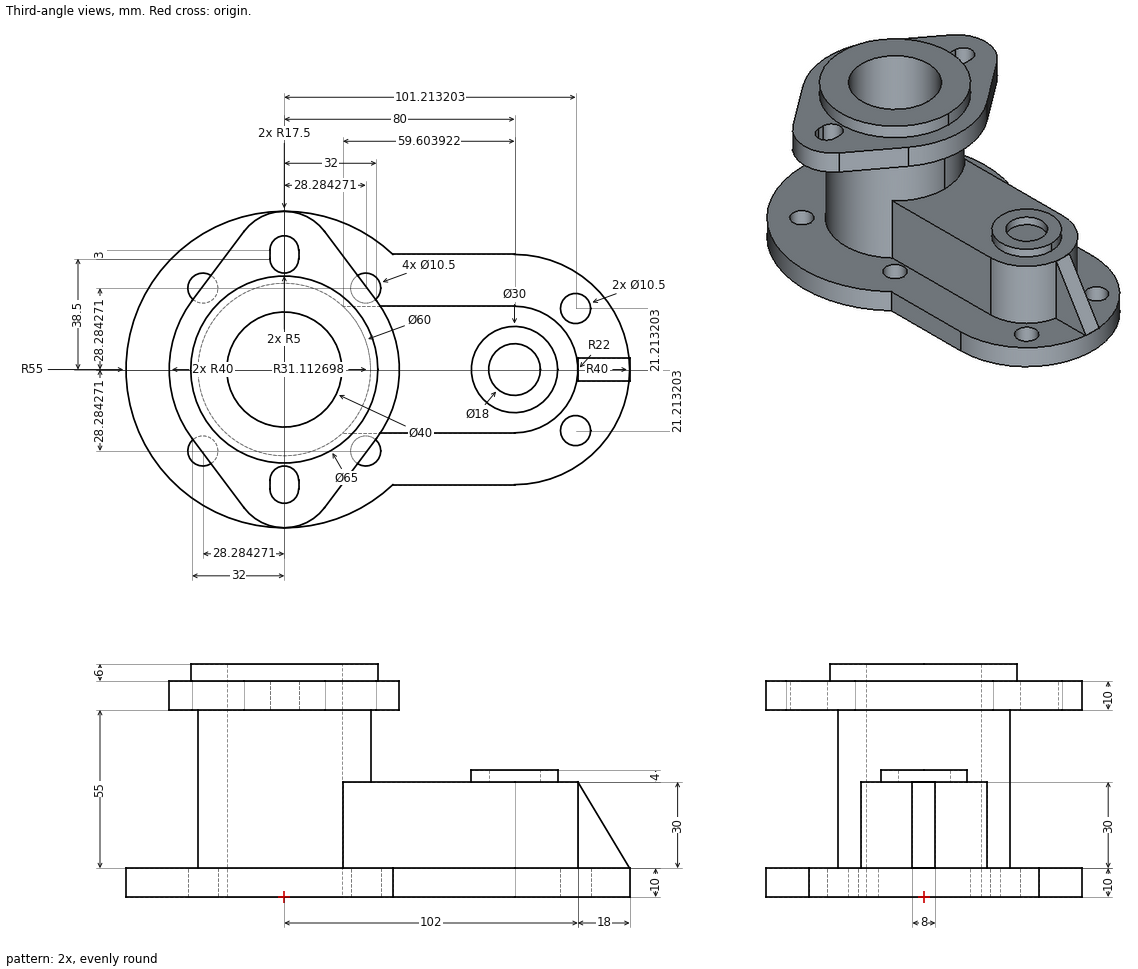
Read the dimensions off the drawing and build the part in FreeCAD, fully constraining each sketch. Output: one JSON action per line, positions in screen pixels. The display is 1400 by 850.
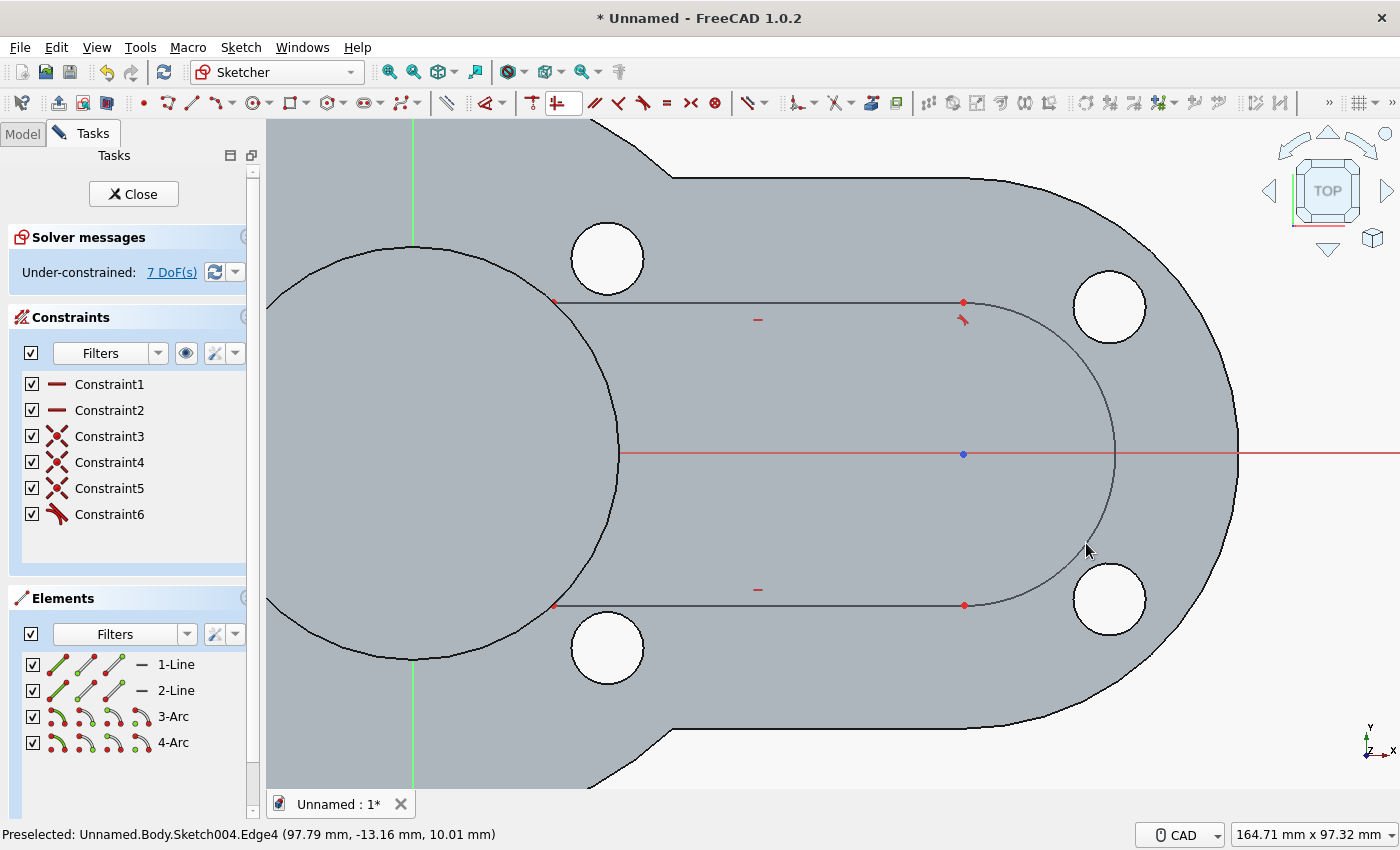
{"action": "left_click", "coordinate": [676, 606]}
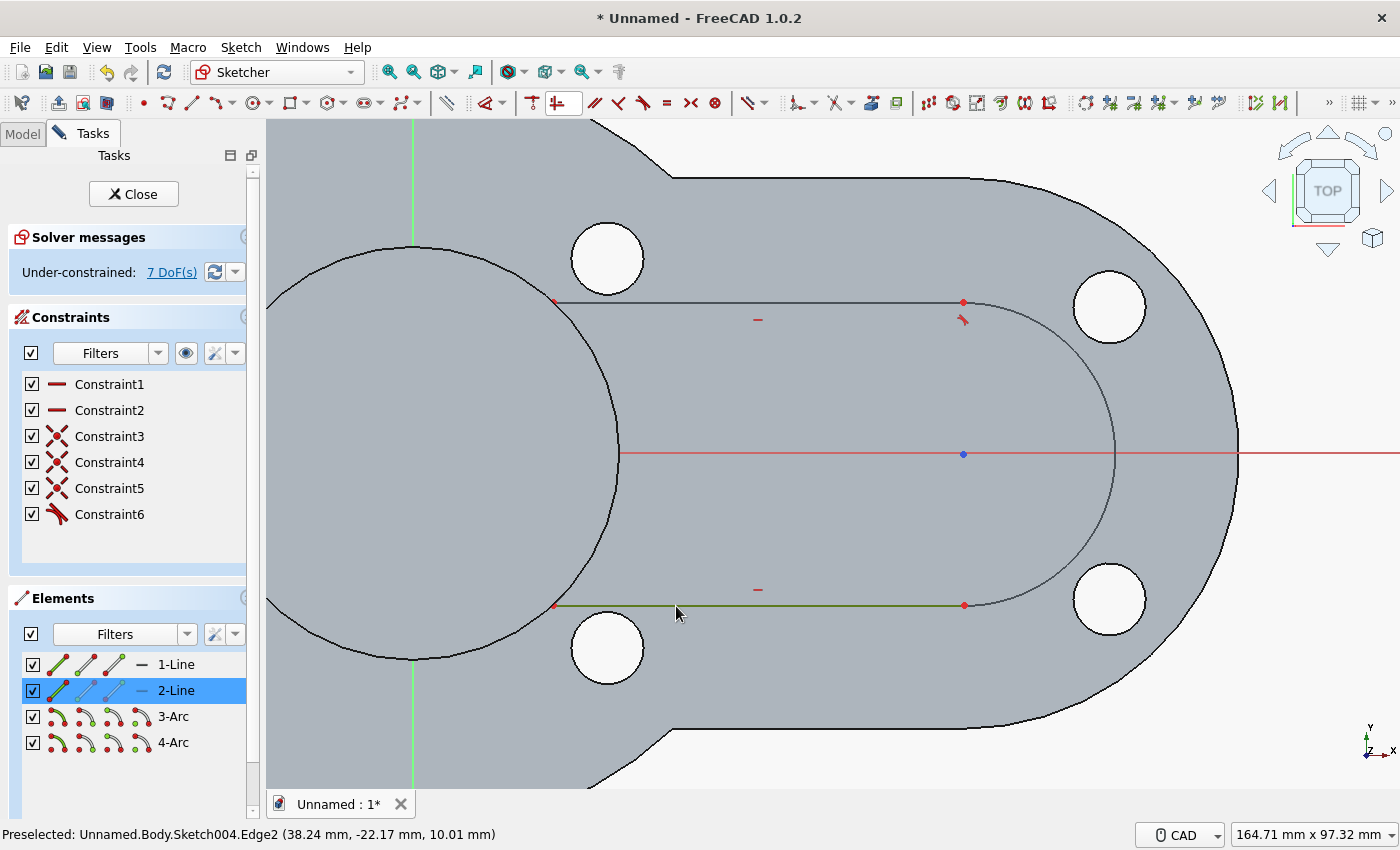
{"action": "left_click", "coordinate": [1086, 543]}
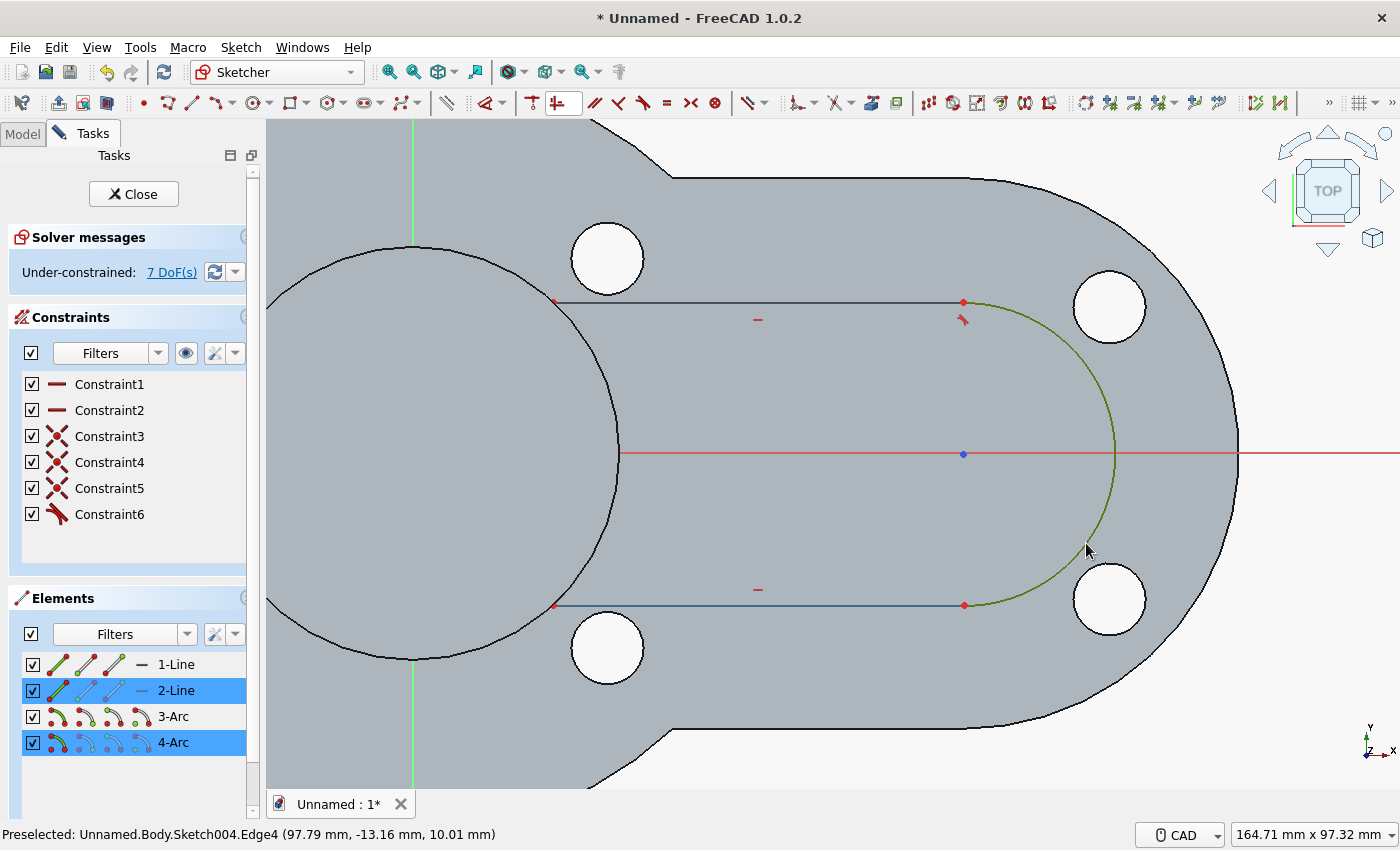
{"action": "left_click", "coordinate": [644, 104]}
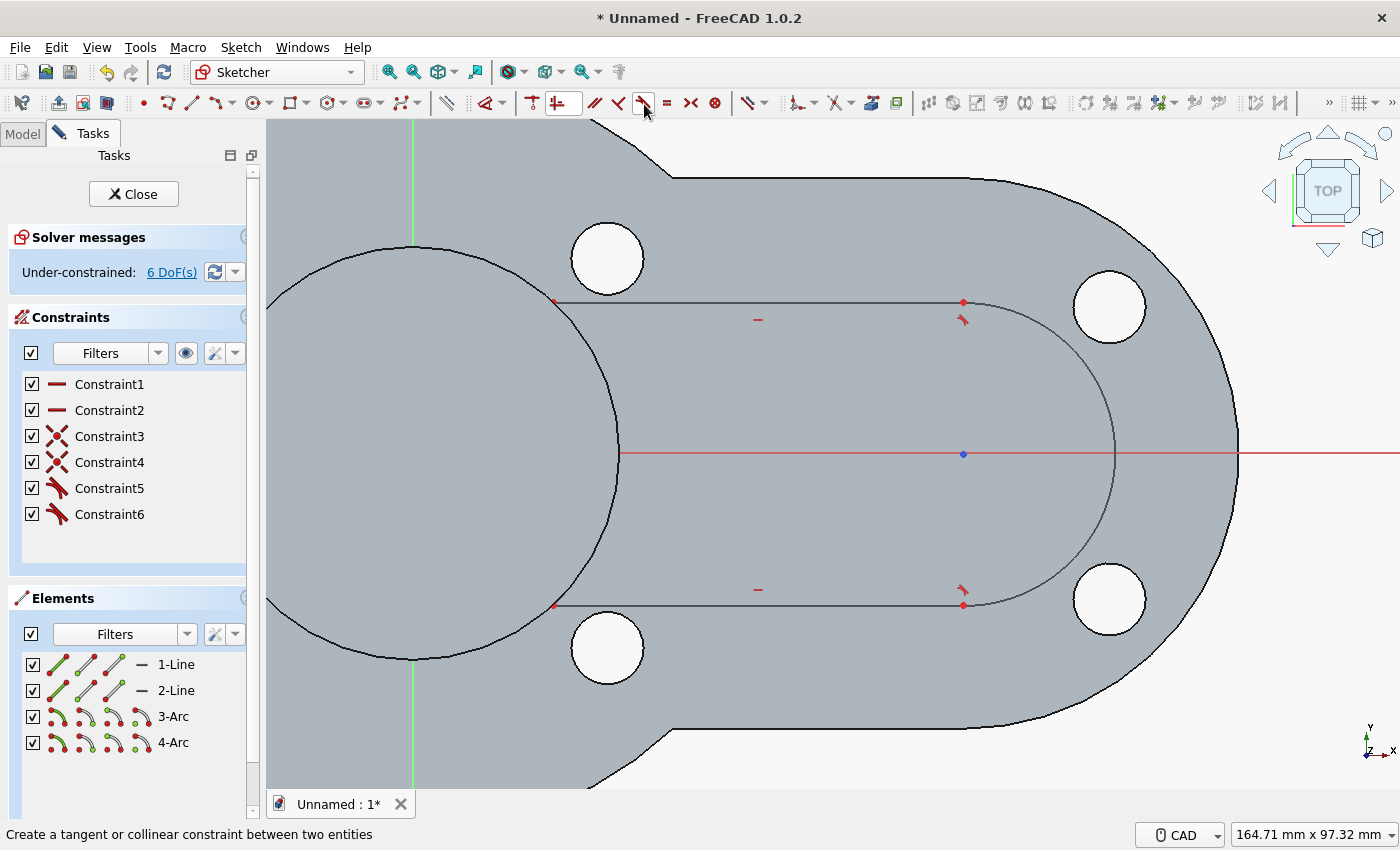
{"action": "left_click", "coordinate": [401, 454]}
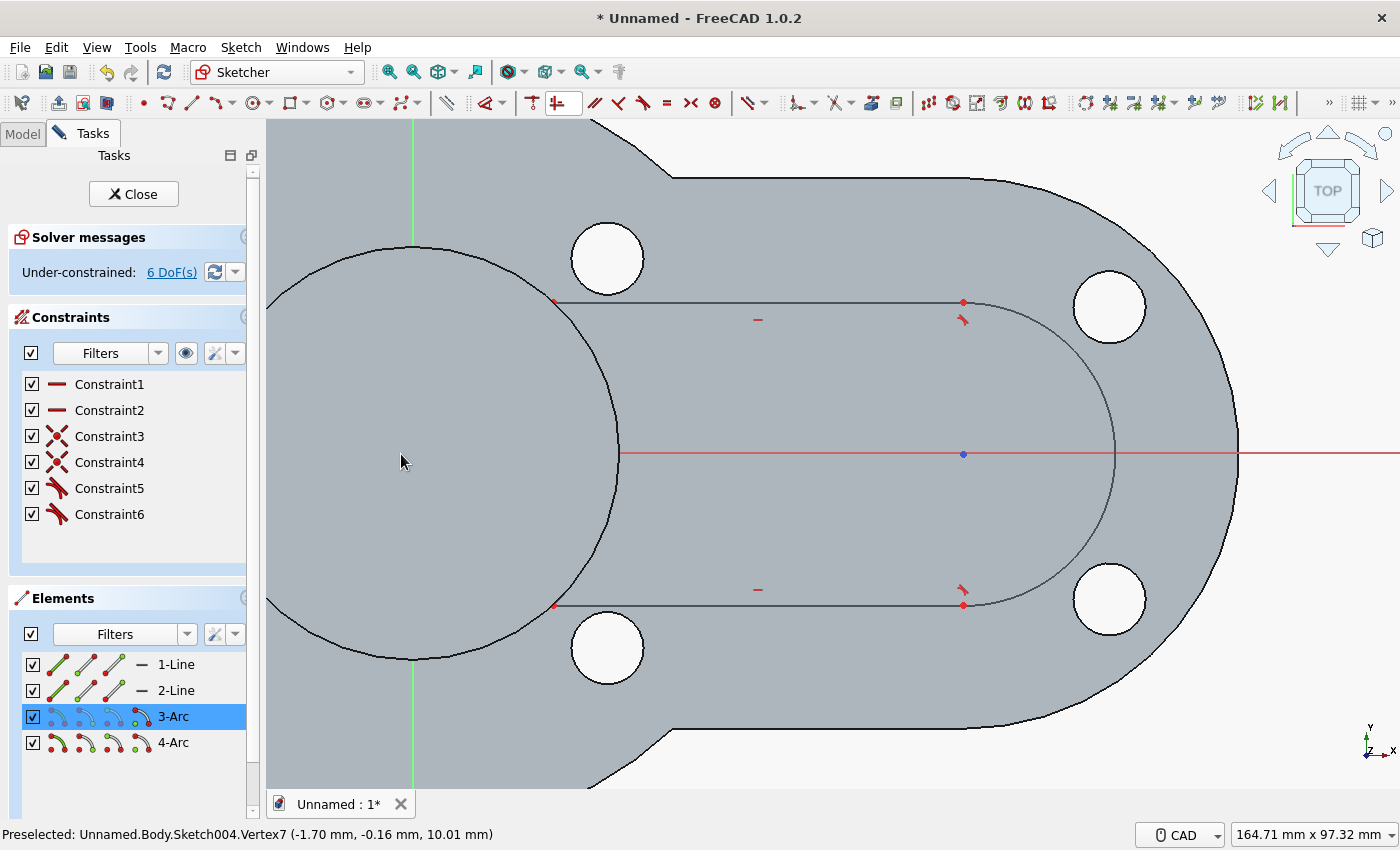
{"action": "left_click", "coordinate": [361, 453]}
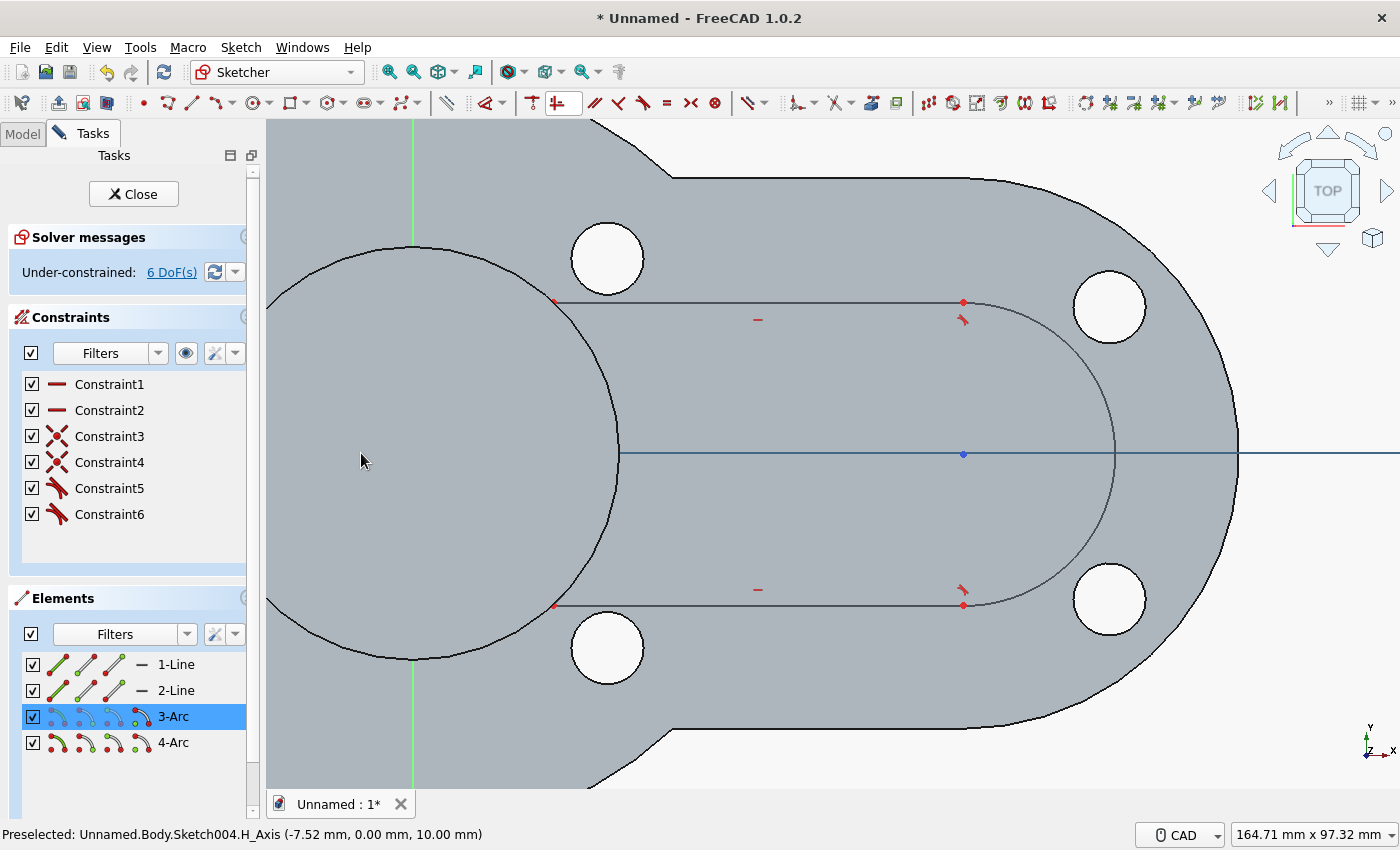
{"action": "key", "text": "c"}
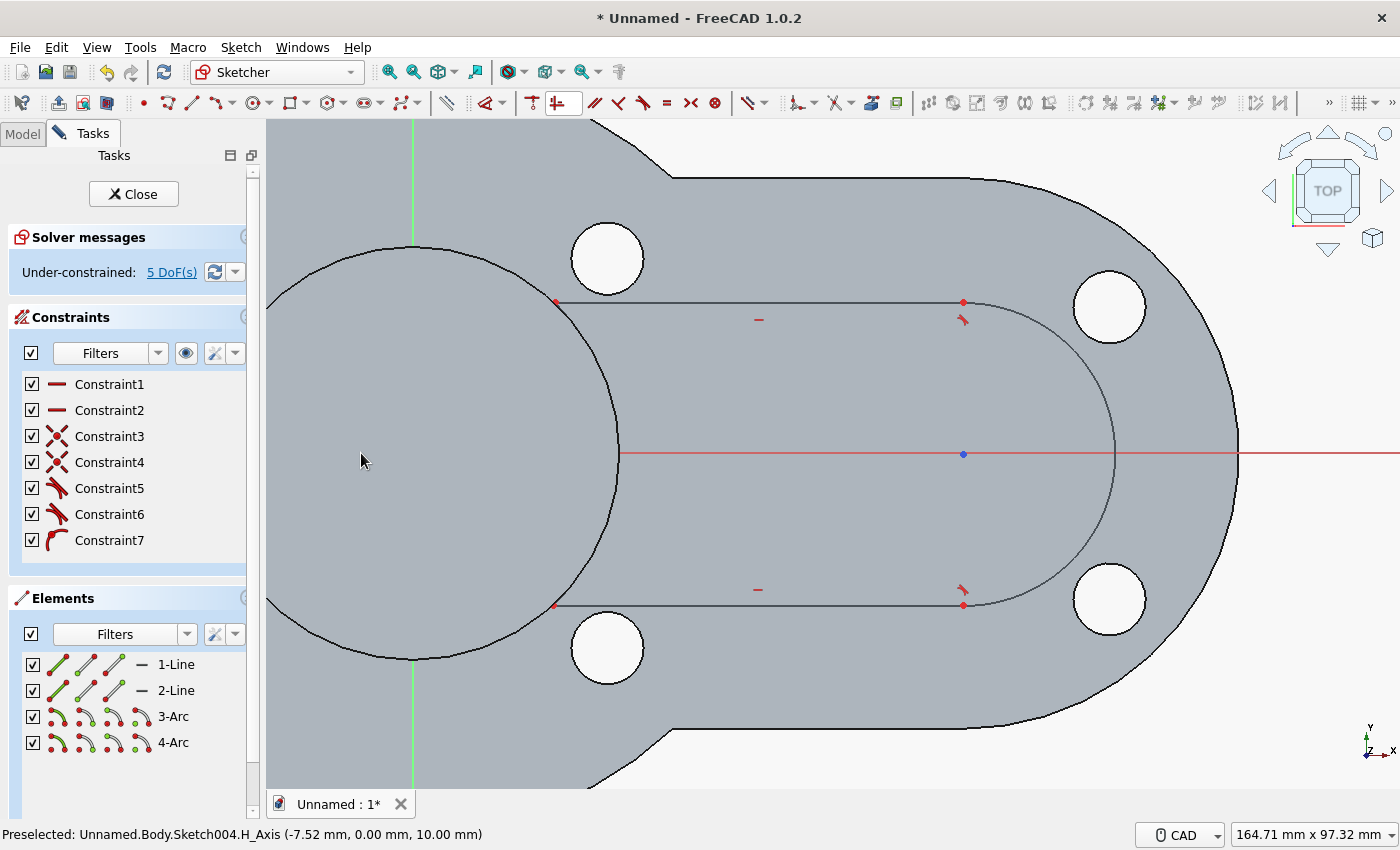
{"action": "left_click", "coordinate": [964, 455]}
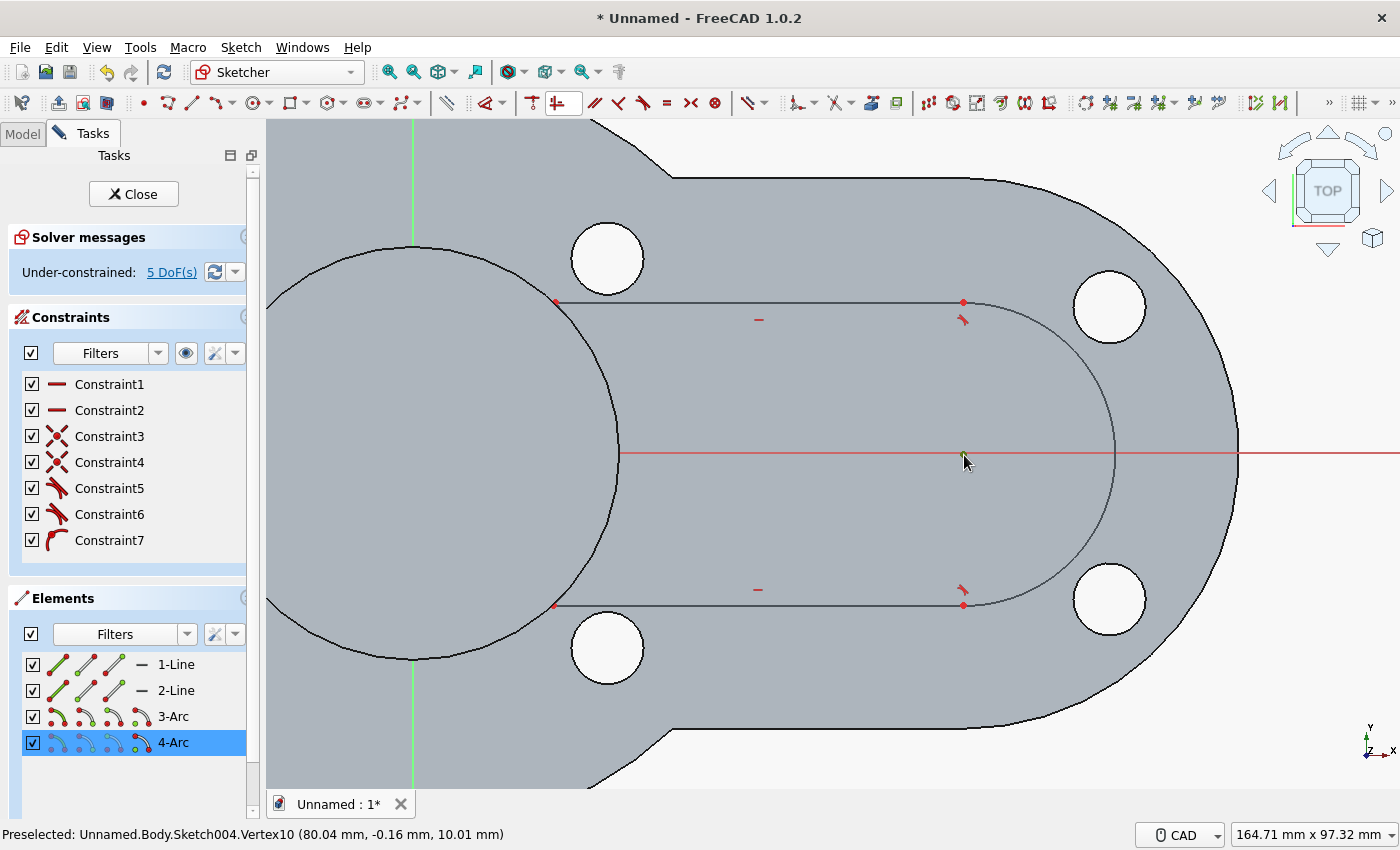
{"action": "left_click", "coordinate": [361, 453]}